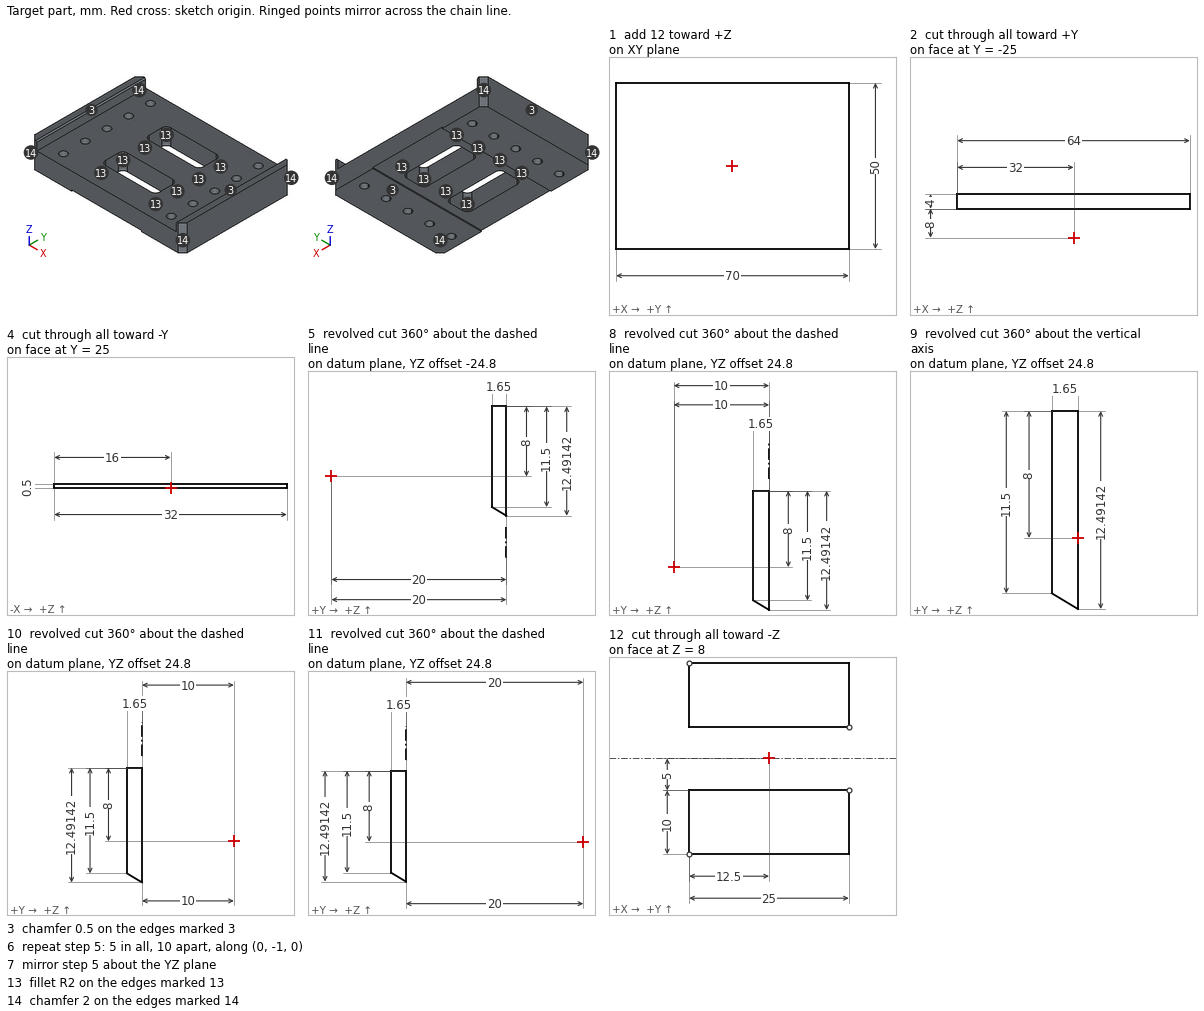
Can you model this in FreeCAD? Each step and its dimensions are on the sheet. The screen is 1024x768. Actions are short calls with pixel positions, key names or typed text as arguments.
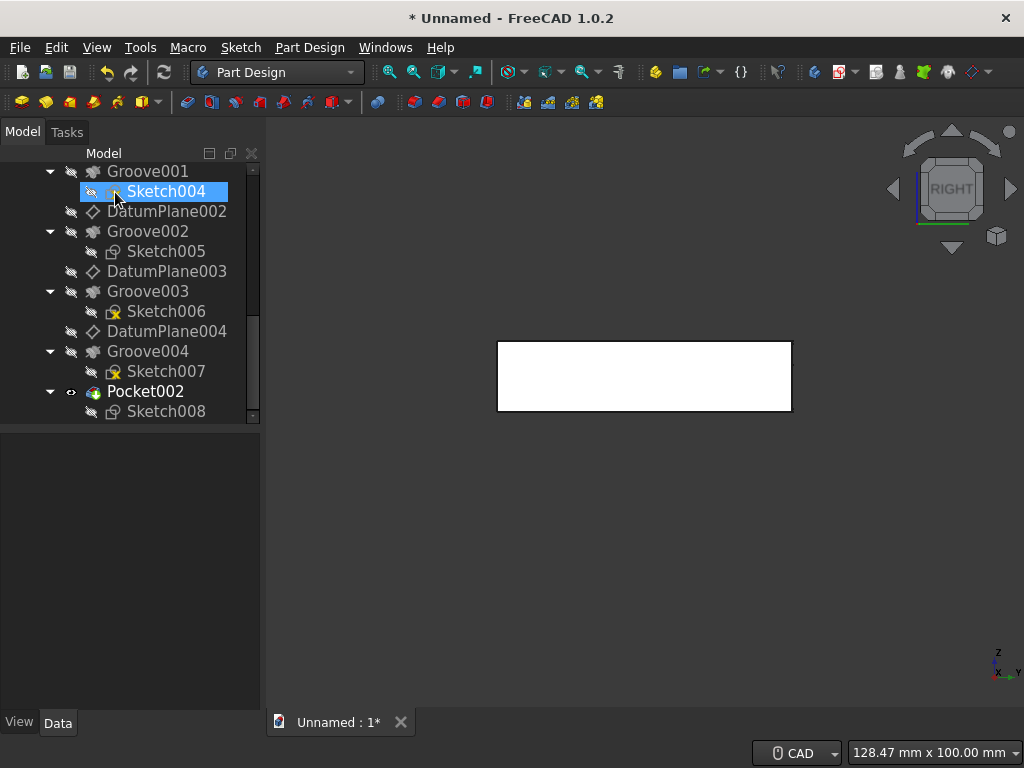
key(v)
key(f)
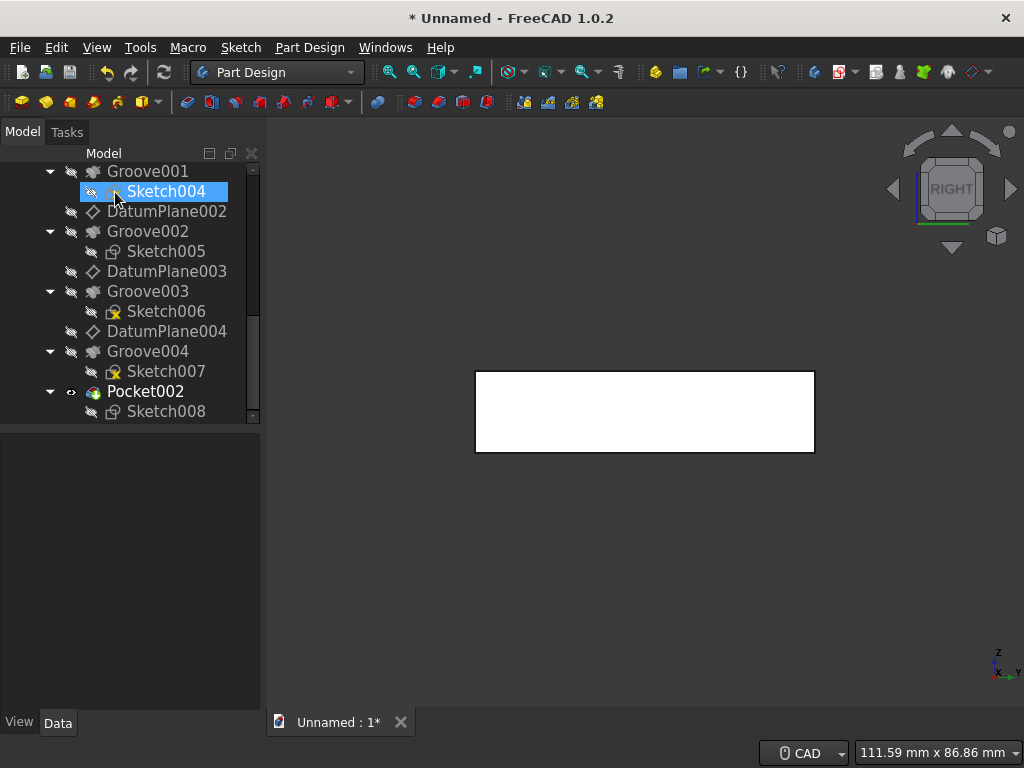
key(5)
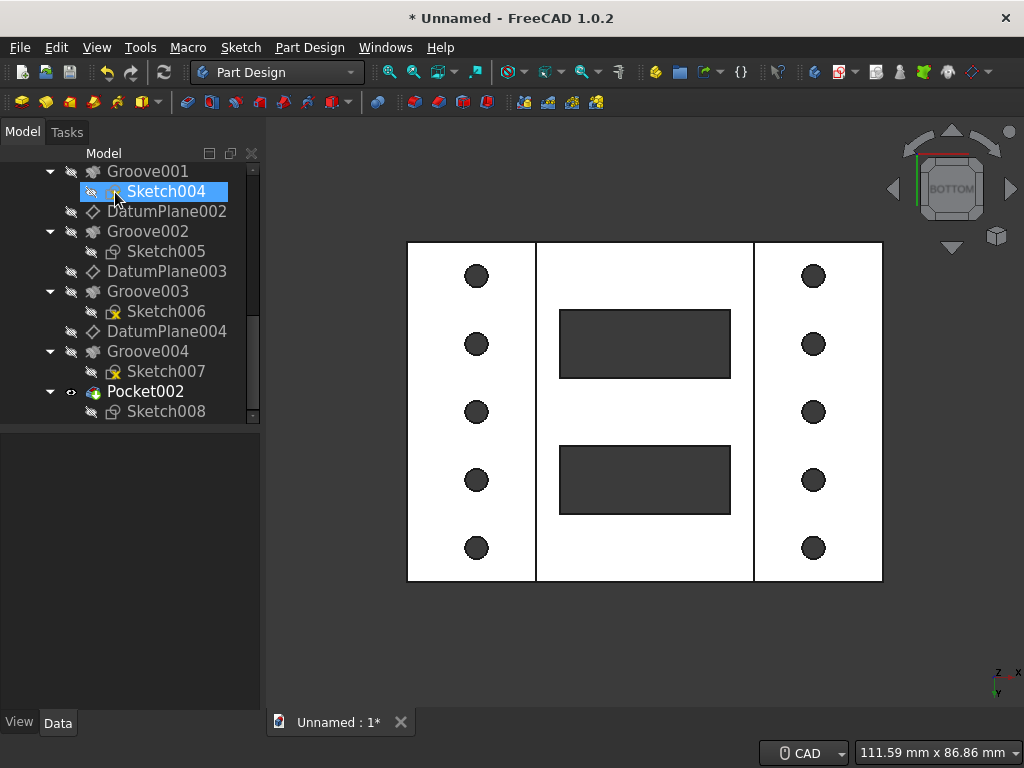
key(4)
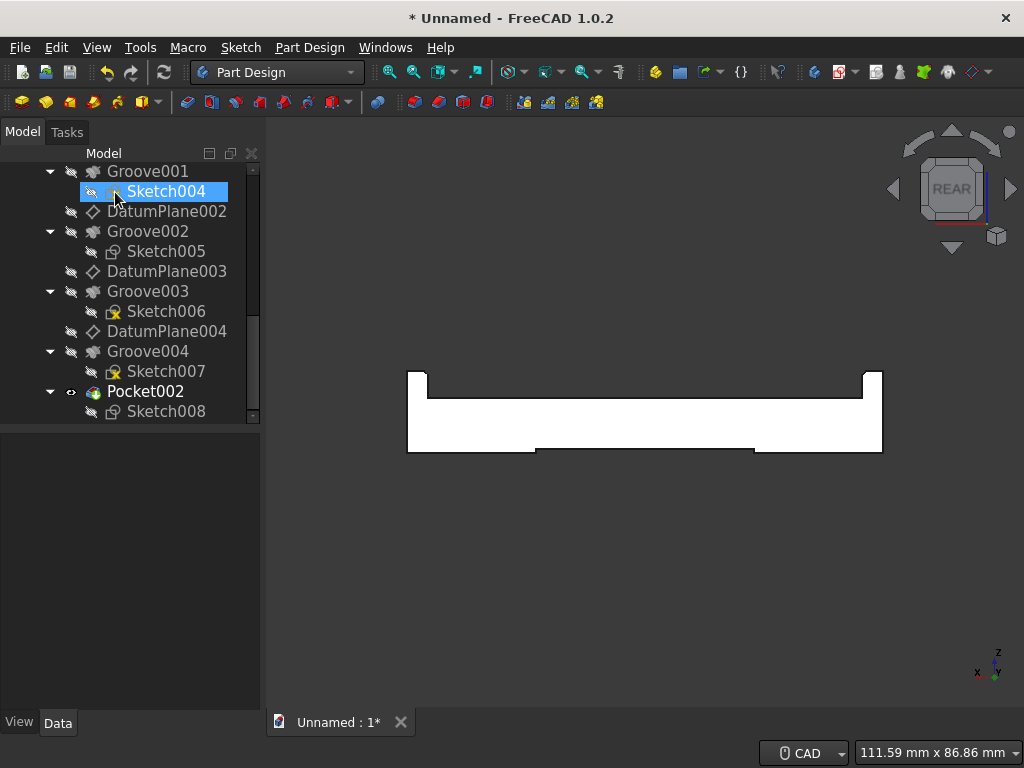
key(6)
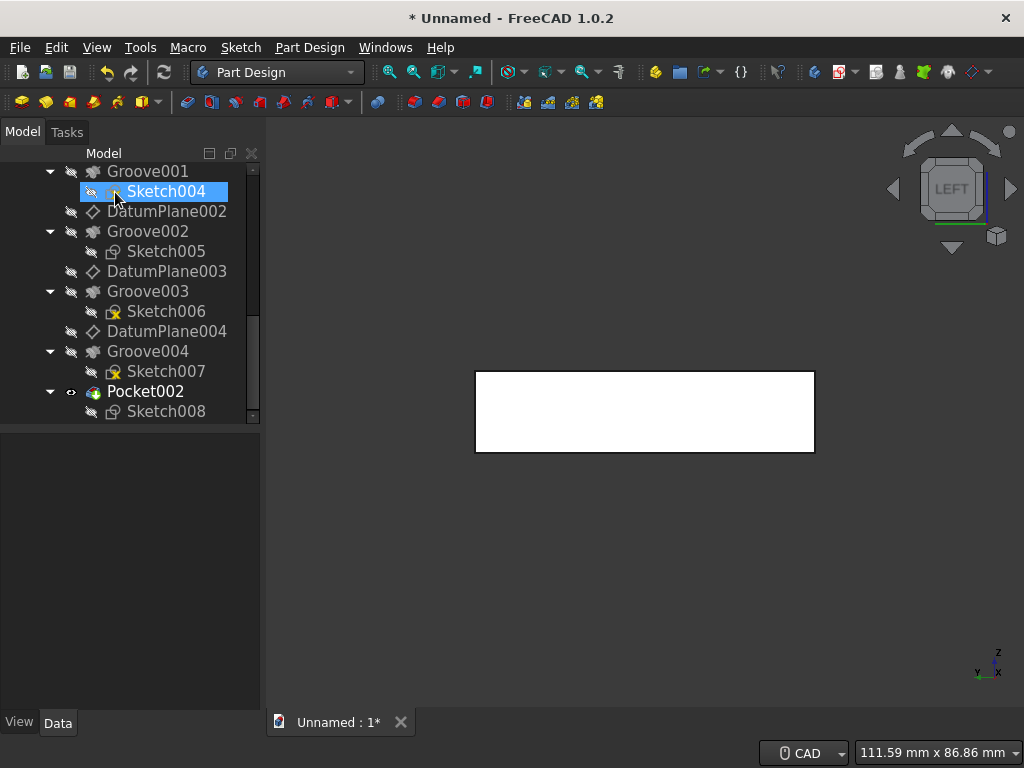
click(390, 72)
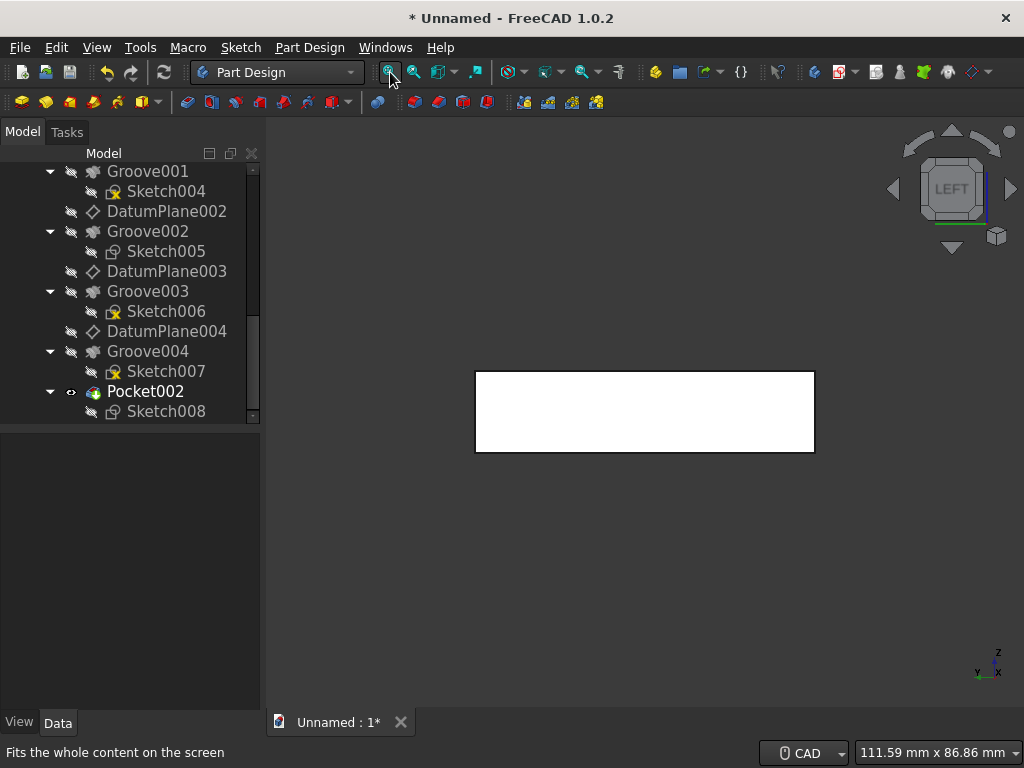
key(v)
key(3)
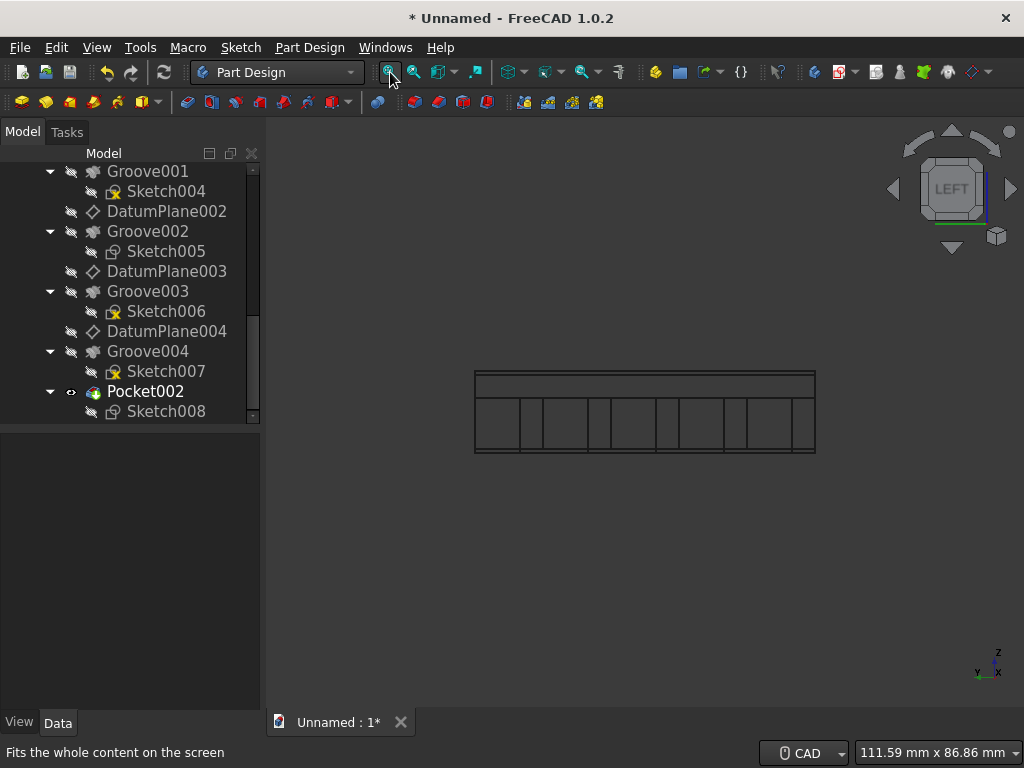
key(0)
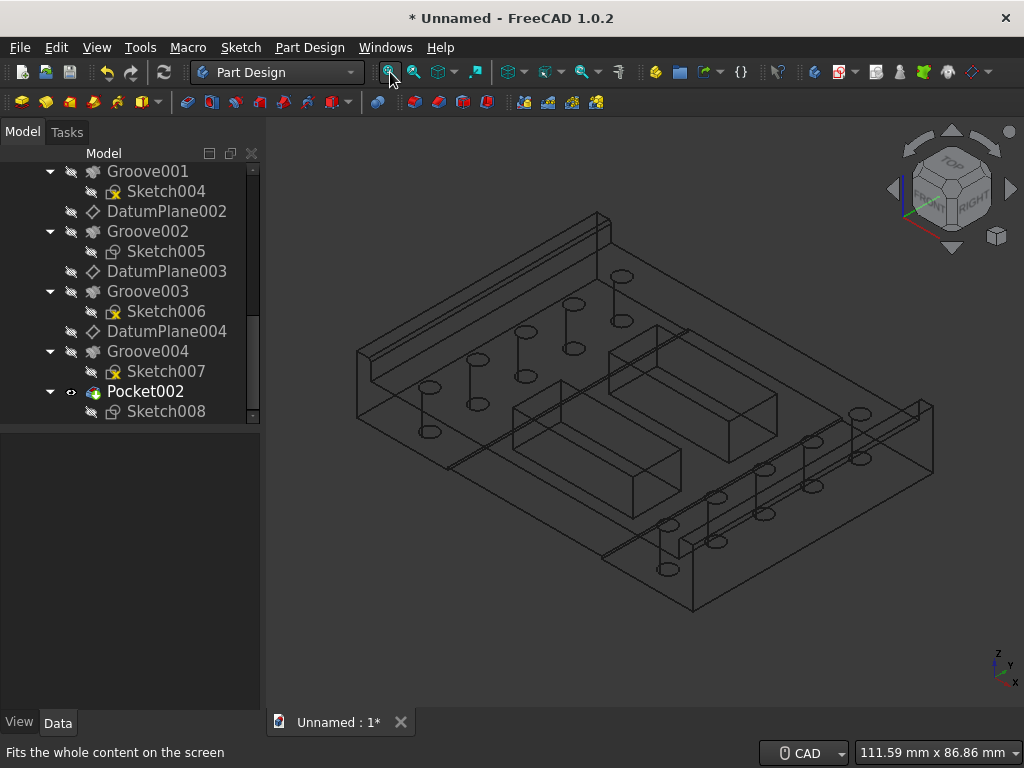
click(513, 428)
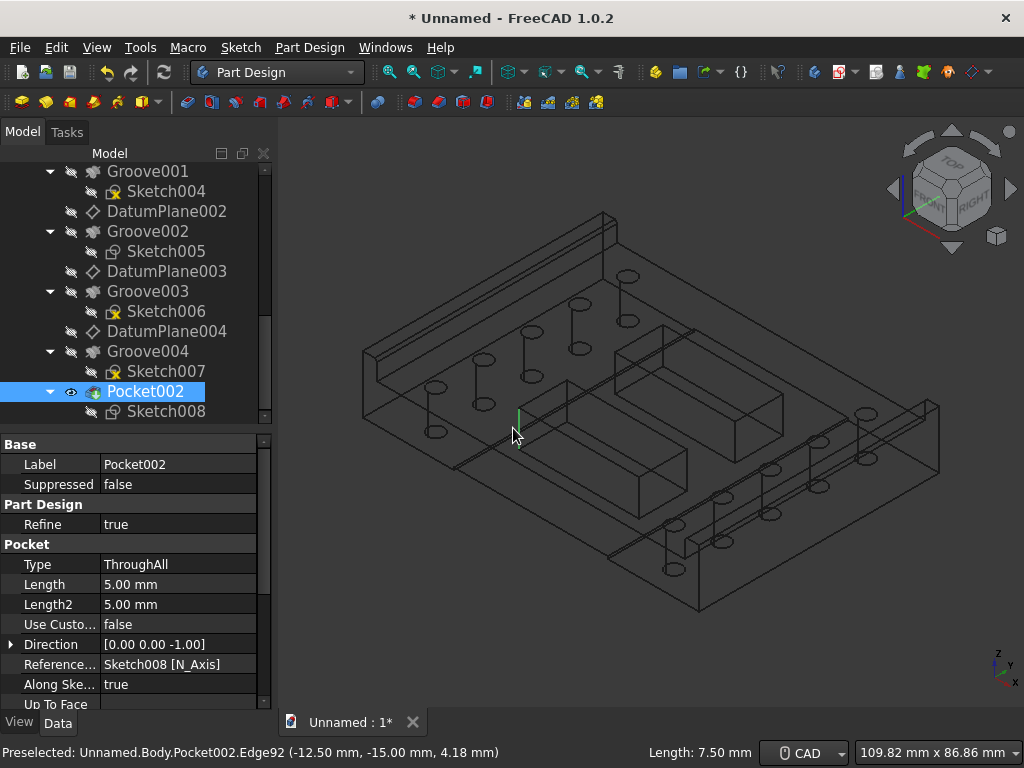
click(567, 400, ctrl)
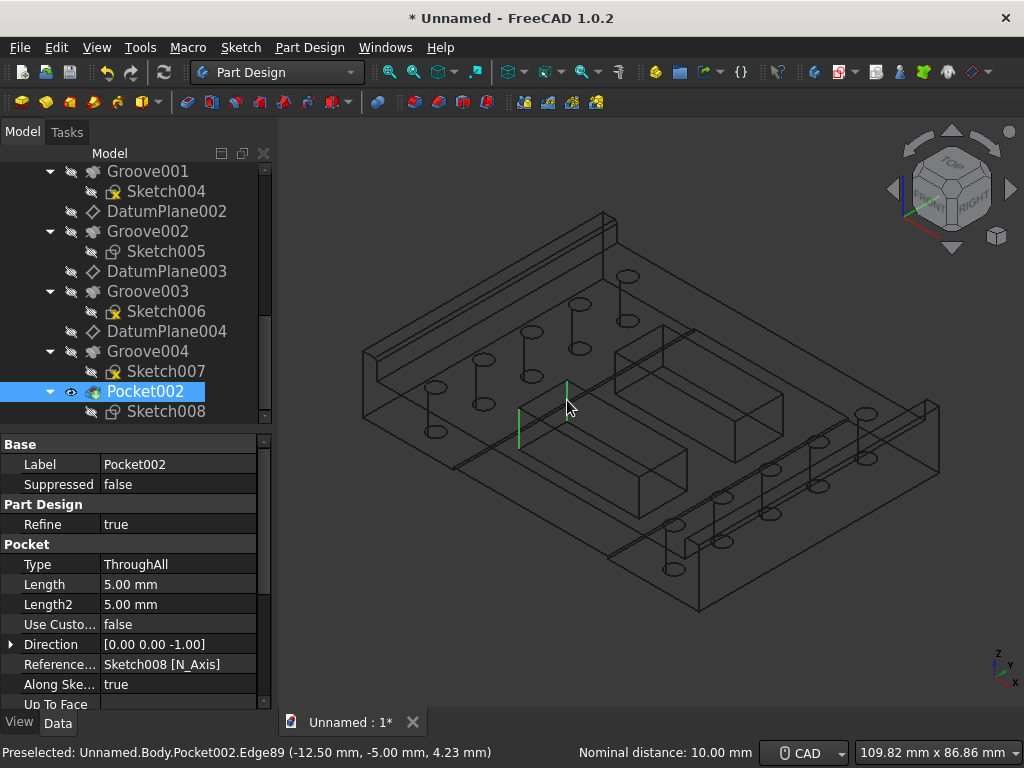
click(687, 469, ctrl)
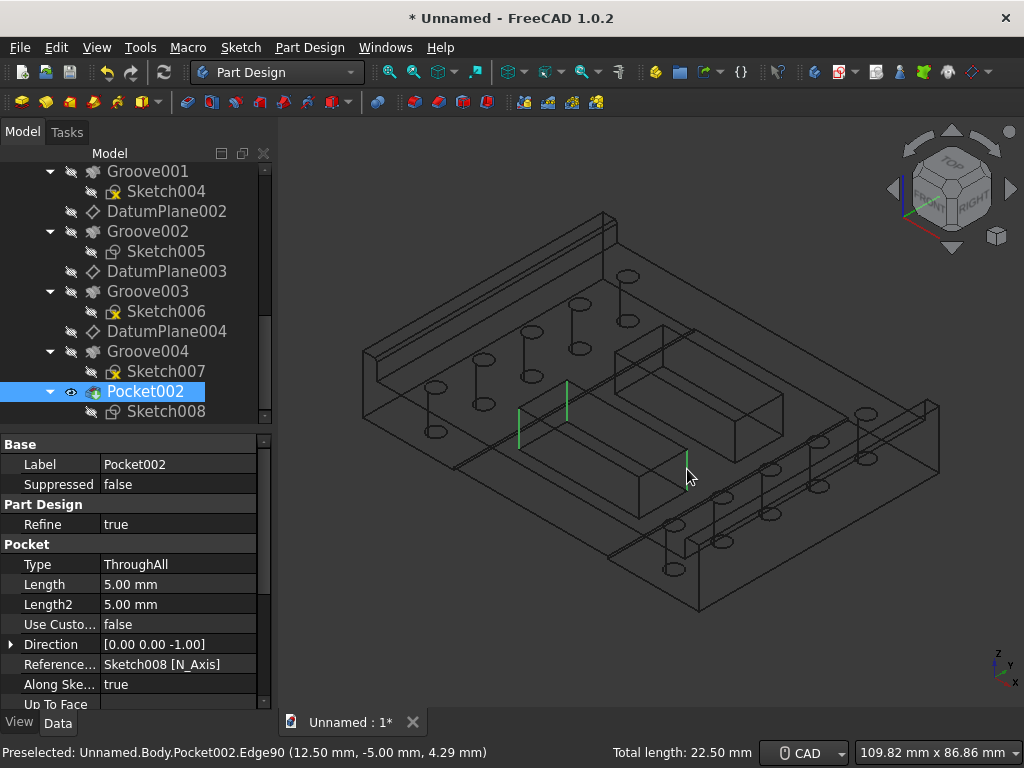
click(639, 497, ctrl)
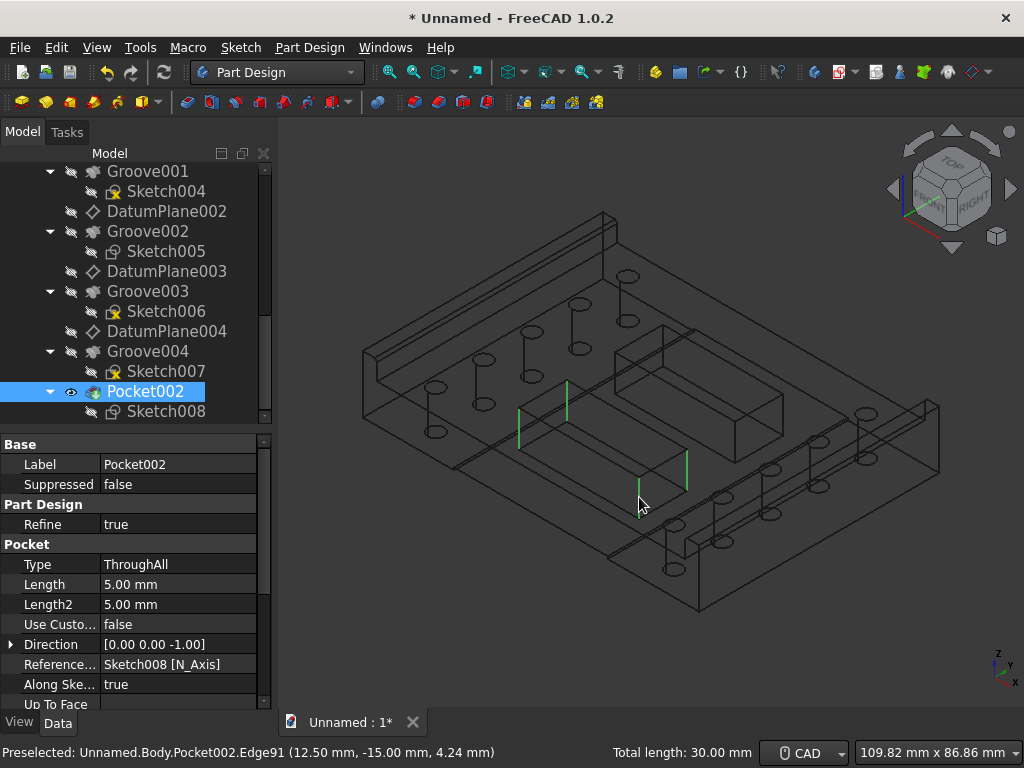
click(735, 442, ctrl)